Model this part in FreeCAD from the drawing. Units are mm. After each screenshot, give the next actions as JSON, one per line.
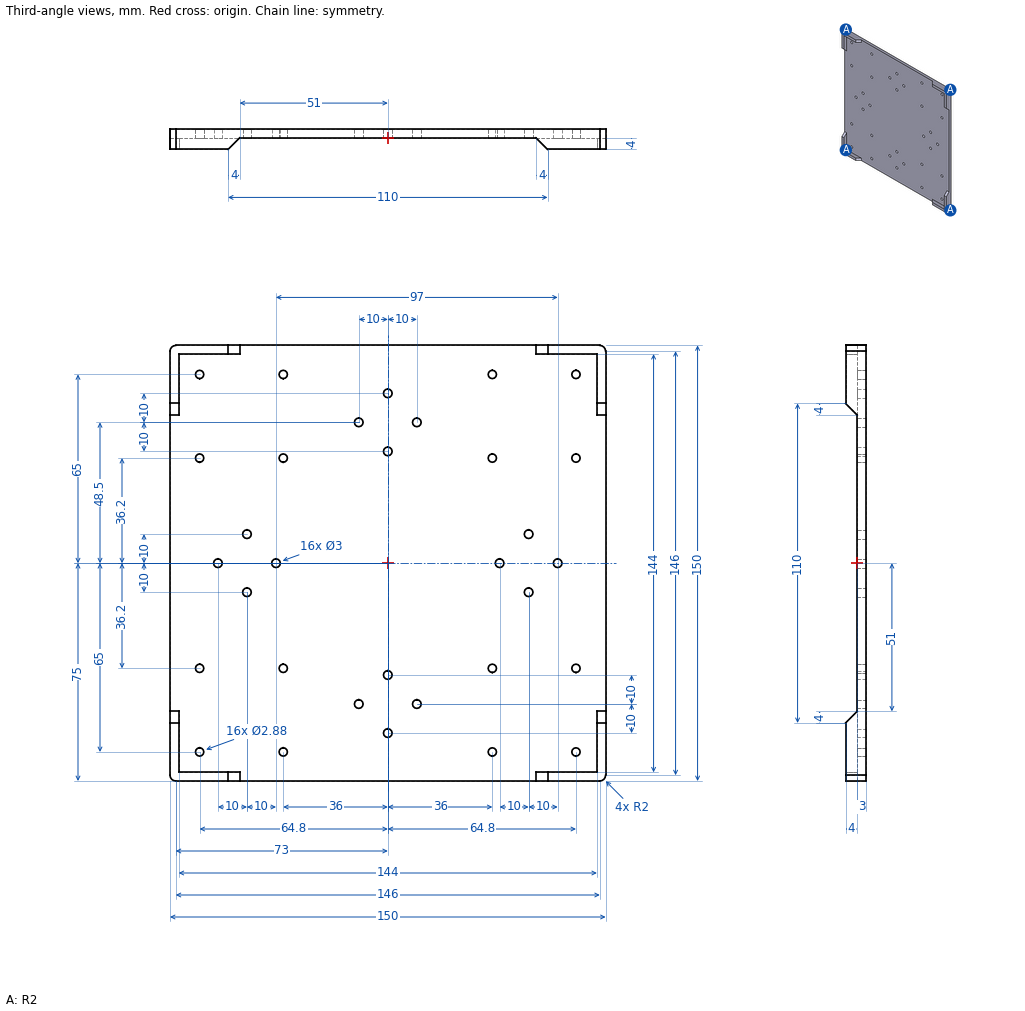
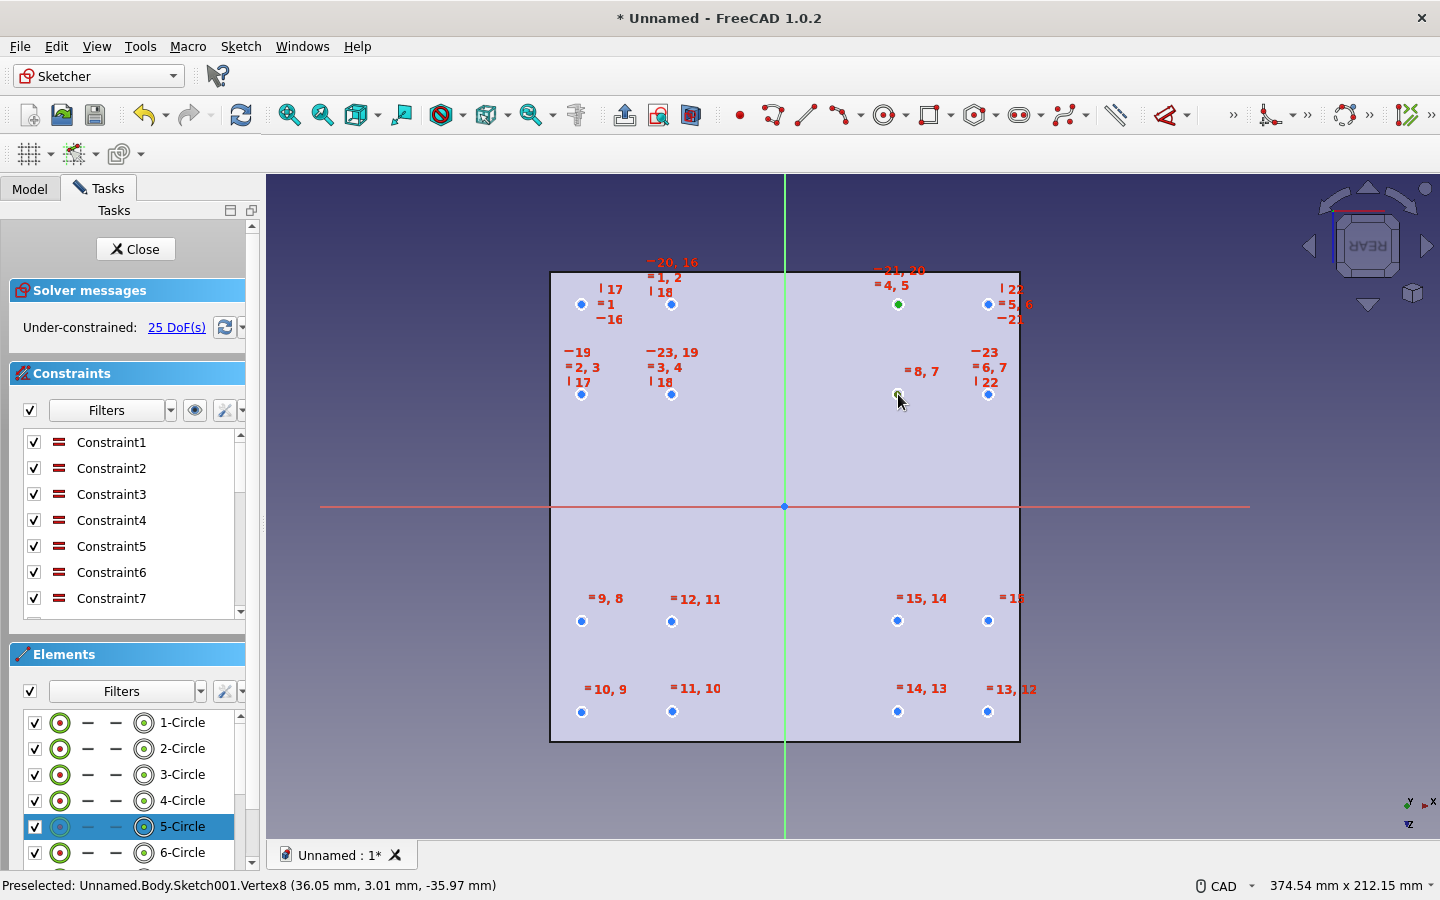
{"action": "key", "text": "v"}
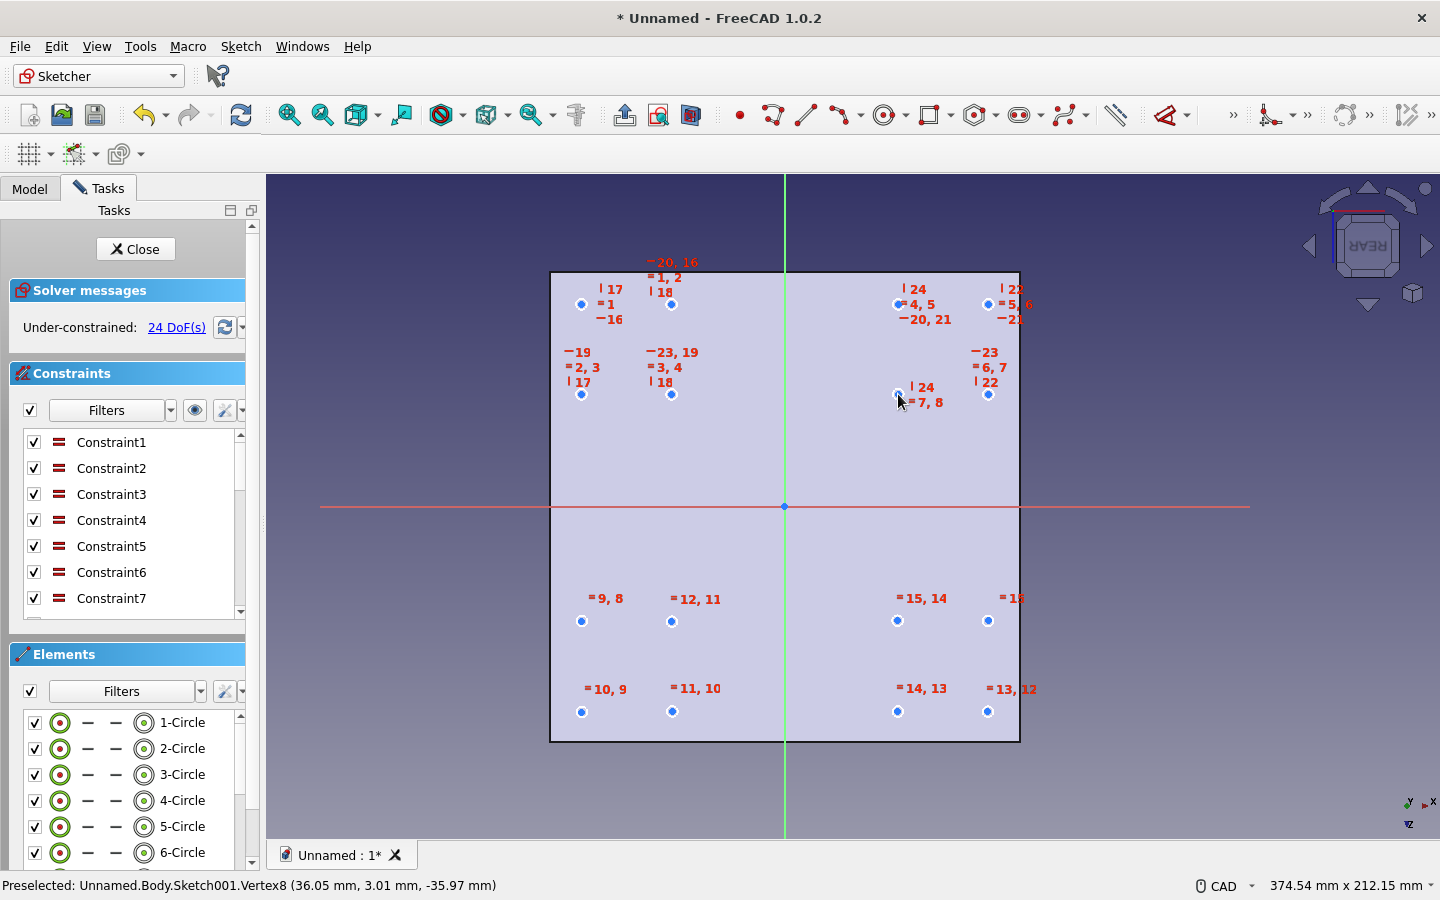
{"action": "left_click", "coordinate": [988, 394]}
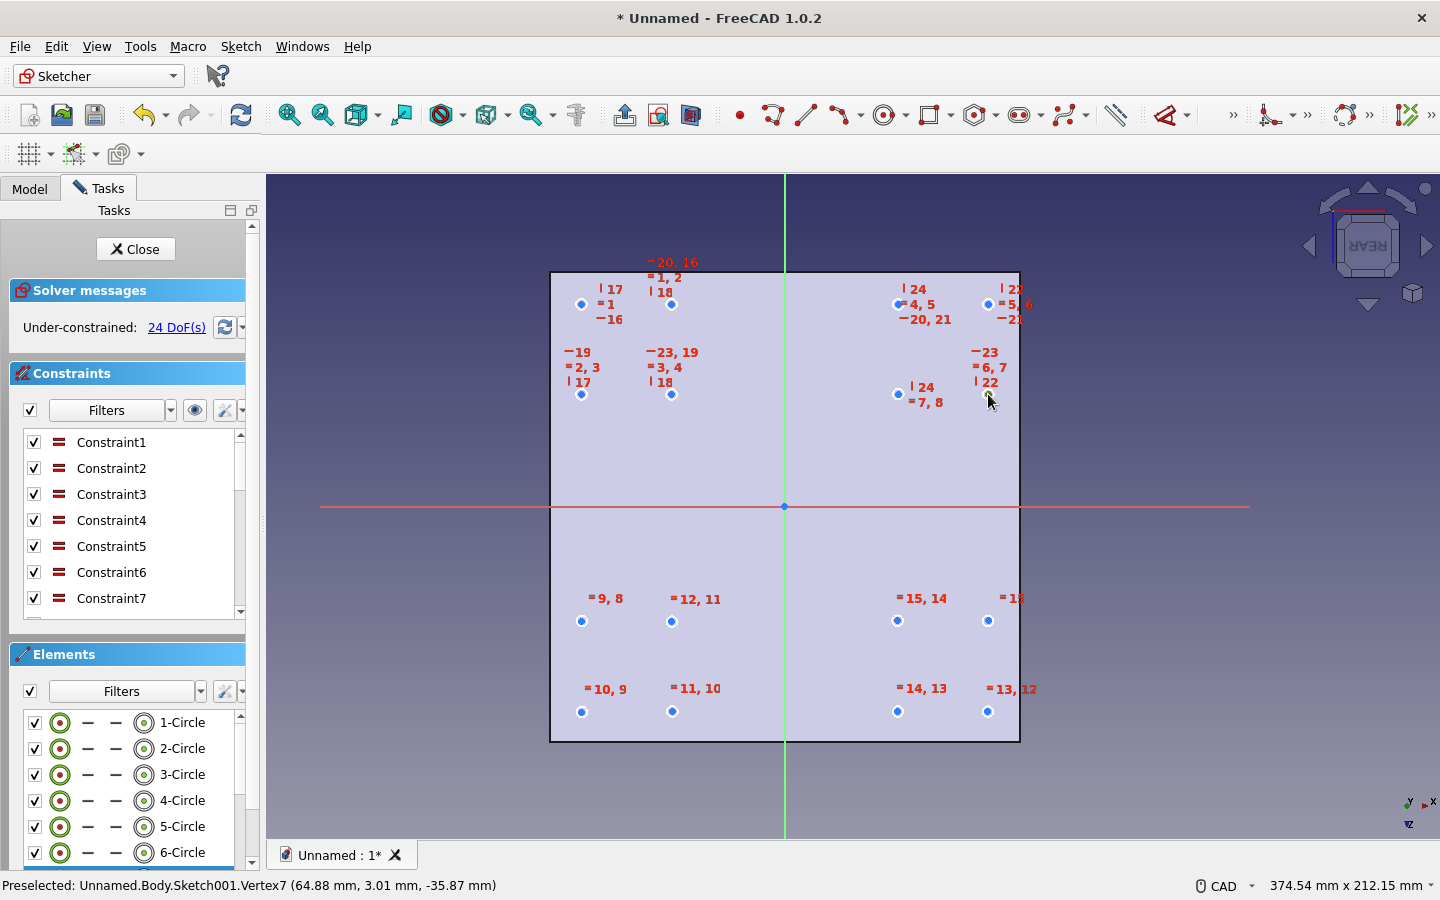
{"action": "left_click", "coordinate": [898, 394]}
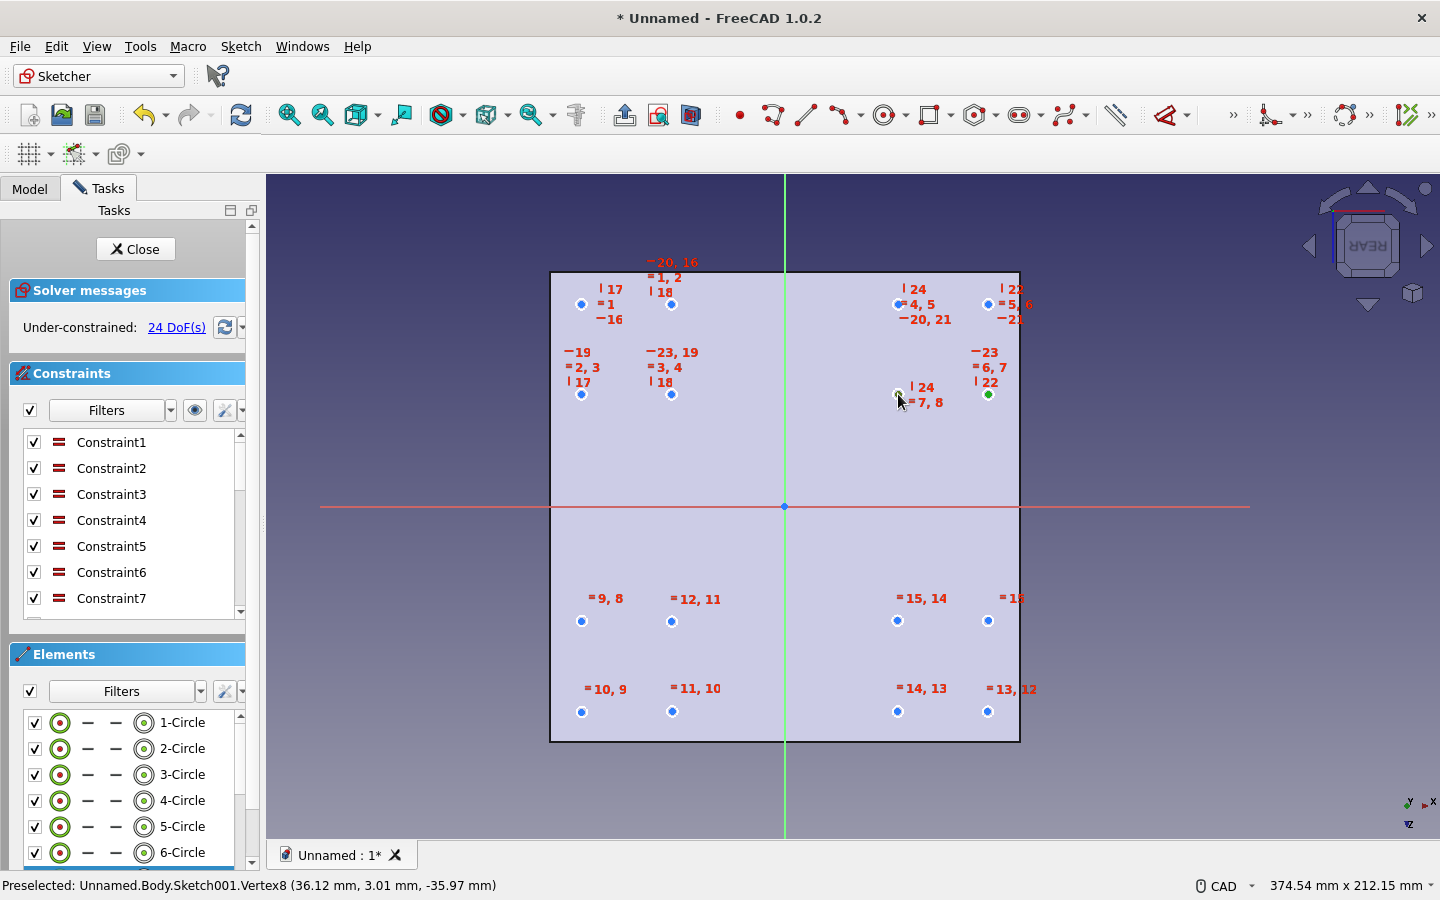
{"action": "key", "text": "h"}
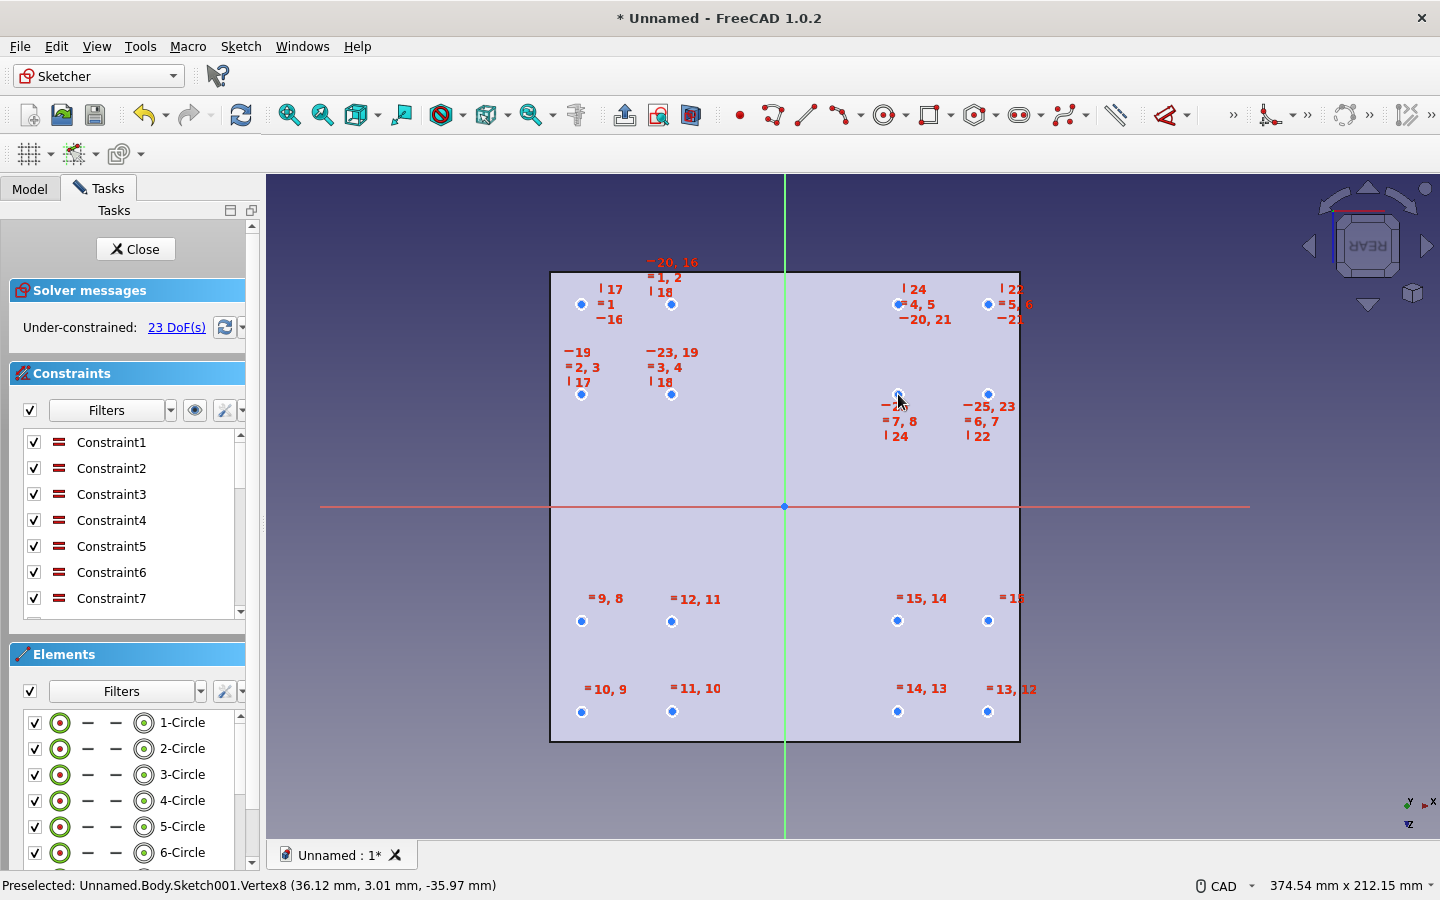
{"action": "left_click", "coordinate": [581, 394]}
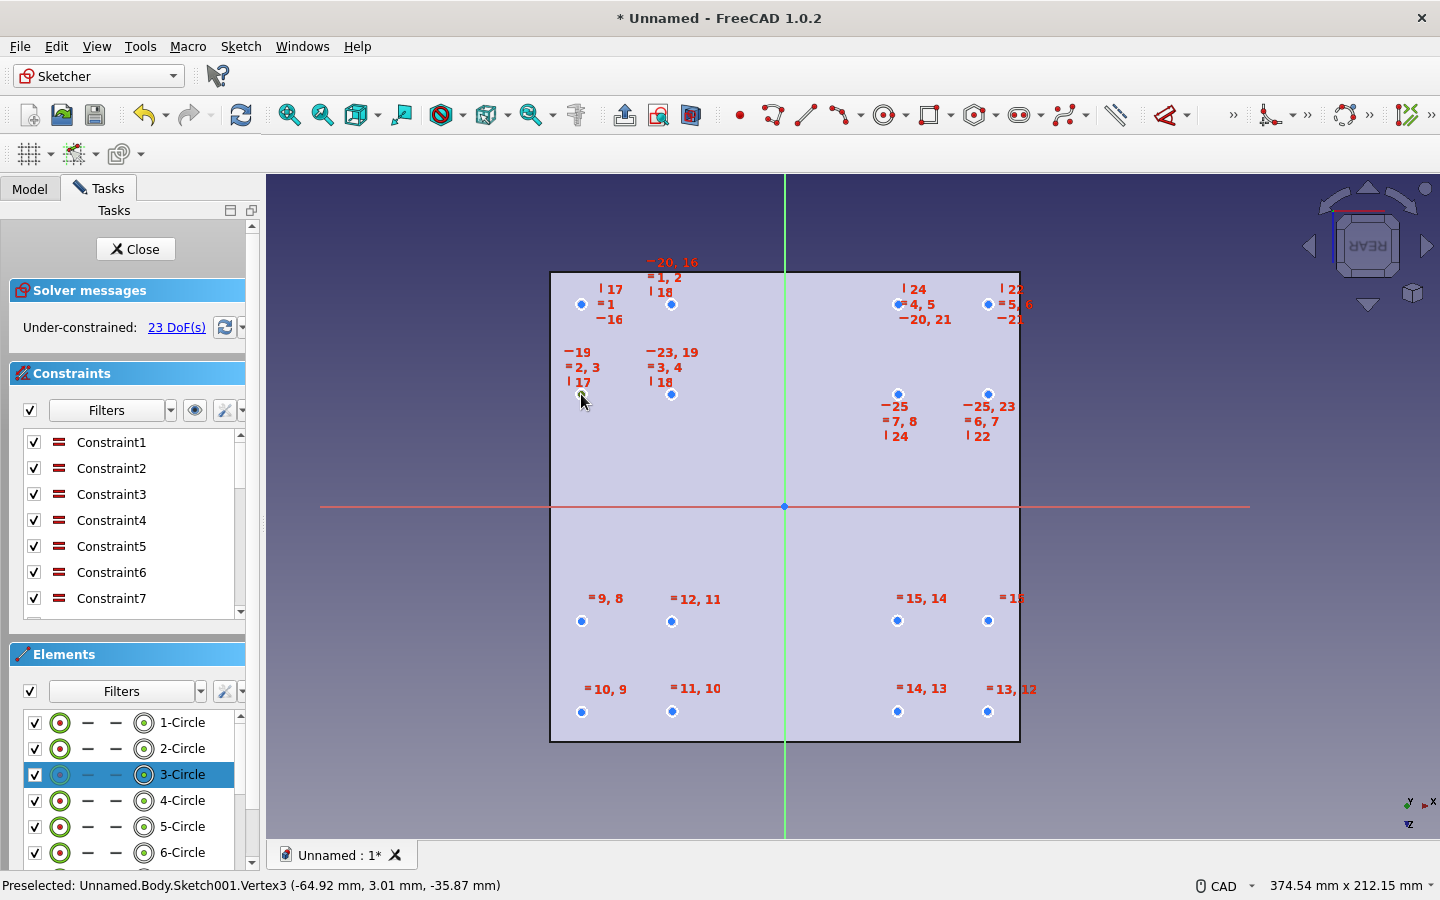
{"action": "left_click", "coordinate": [582, 621]}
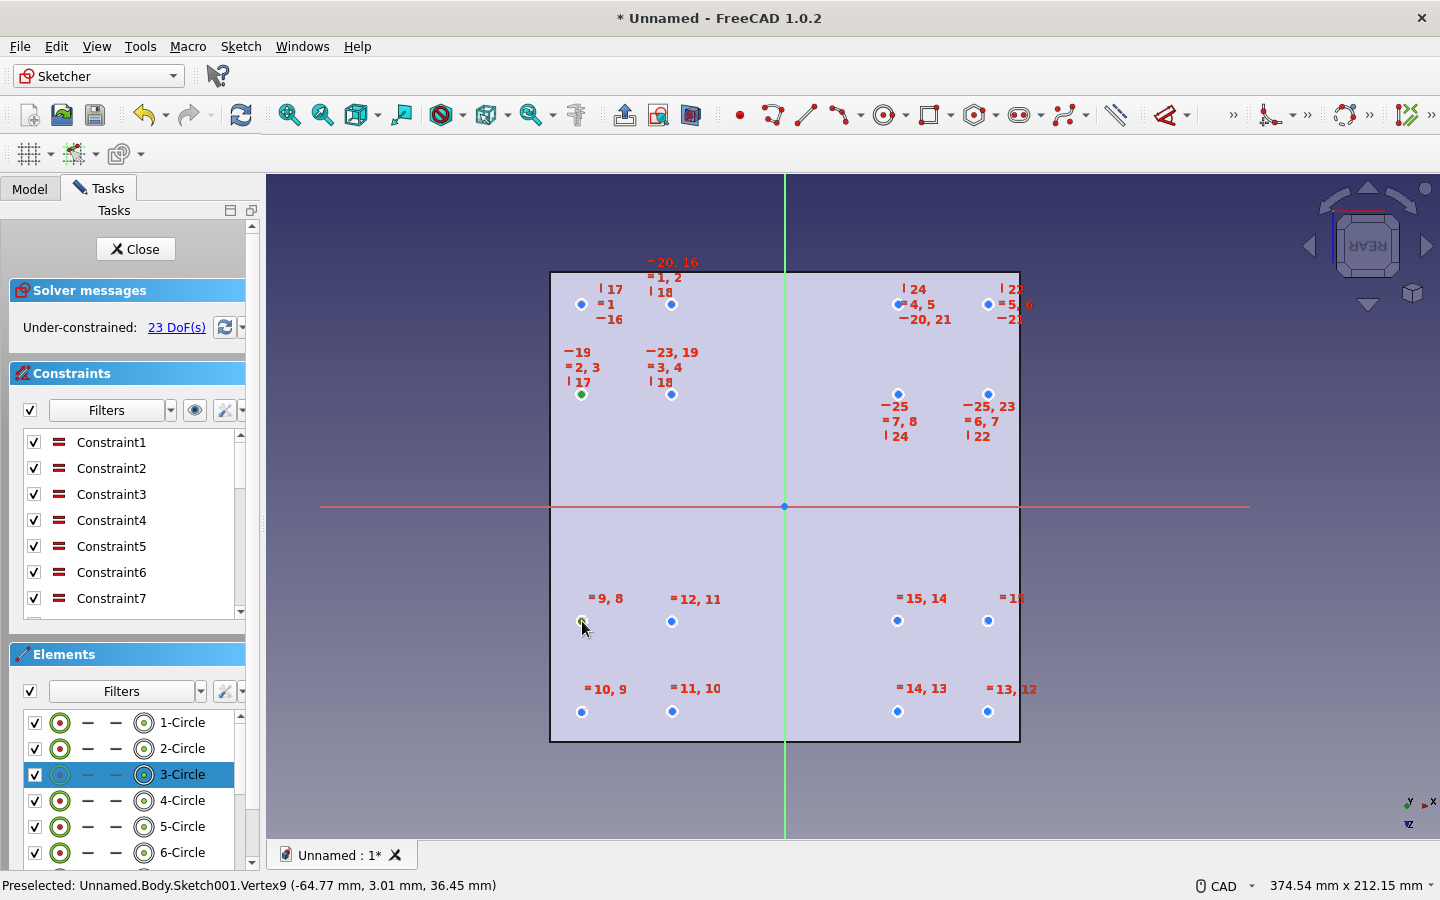
{"action": "key", "text": "v"}